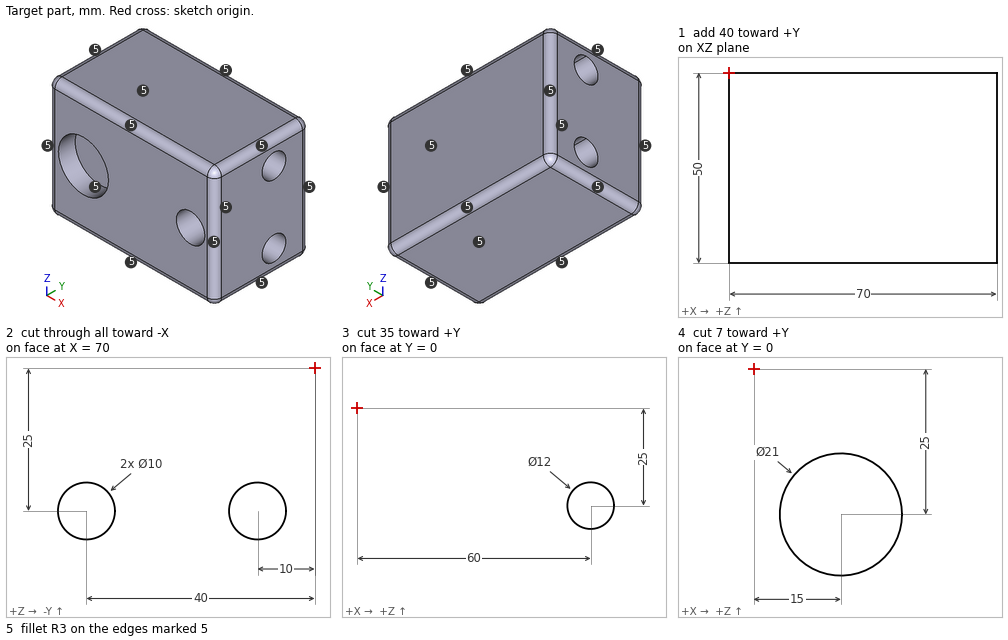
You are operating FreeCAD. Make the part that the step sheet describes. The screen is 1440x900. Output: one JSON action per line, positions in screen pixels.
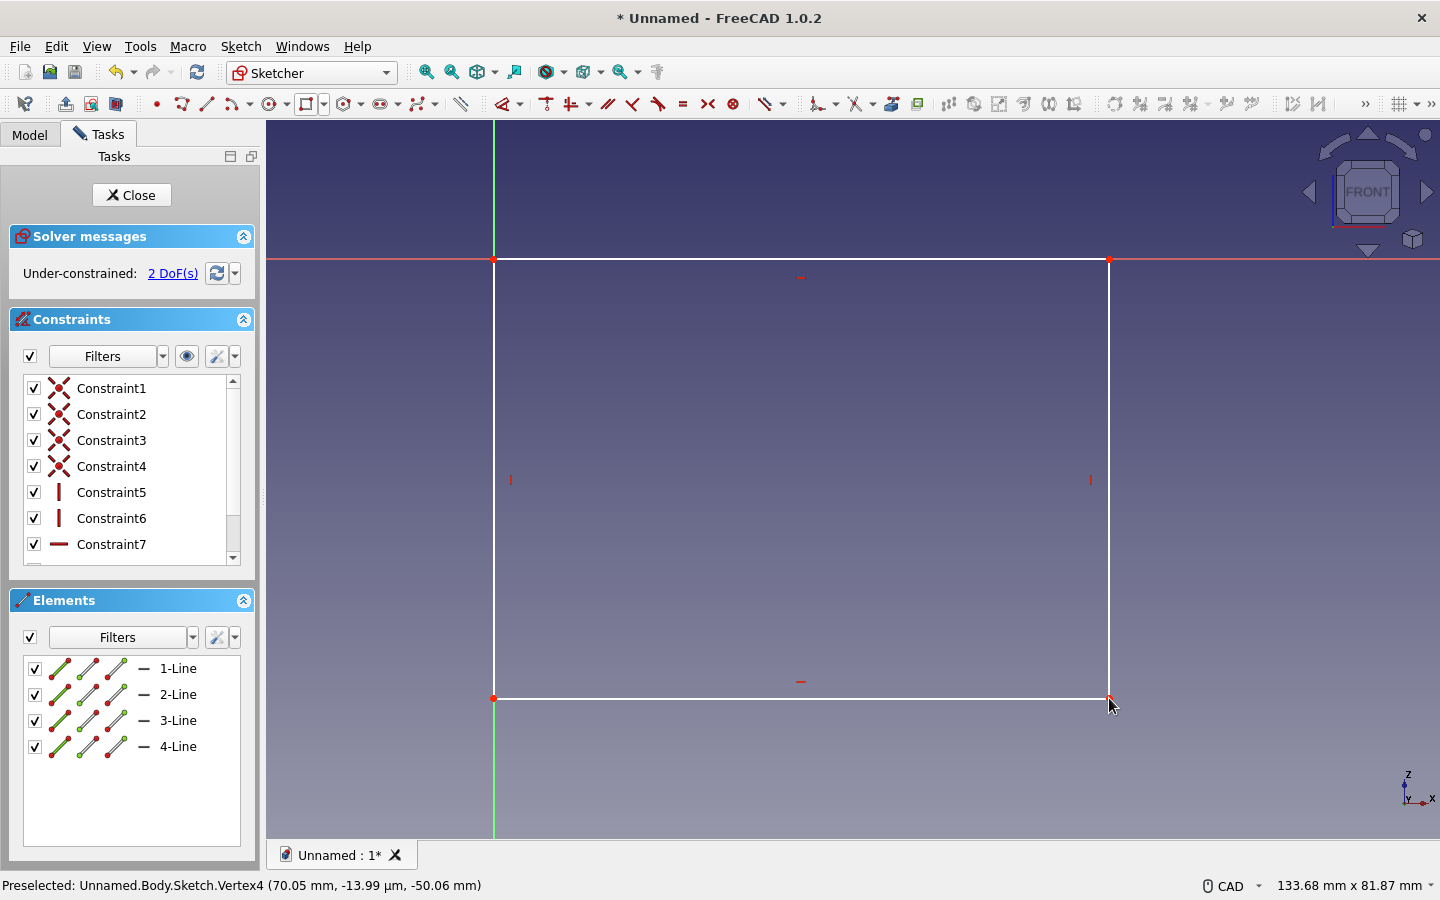
{"action": "left_click", "coordinate": [494, 391]}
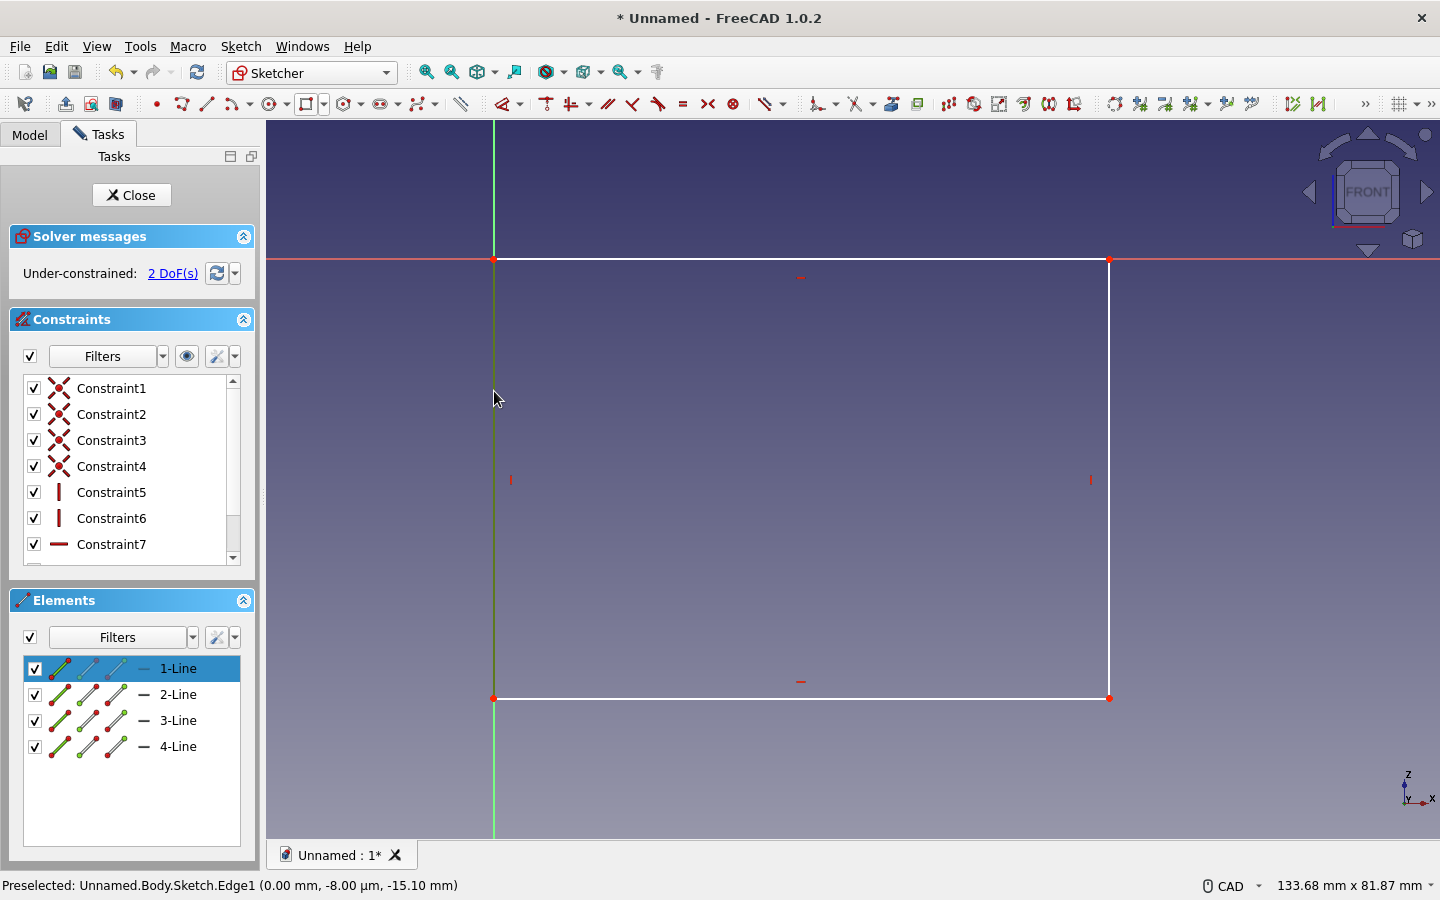
{"action": "key", "text": "i"}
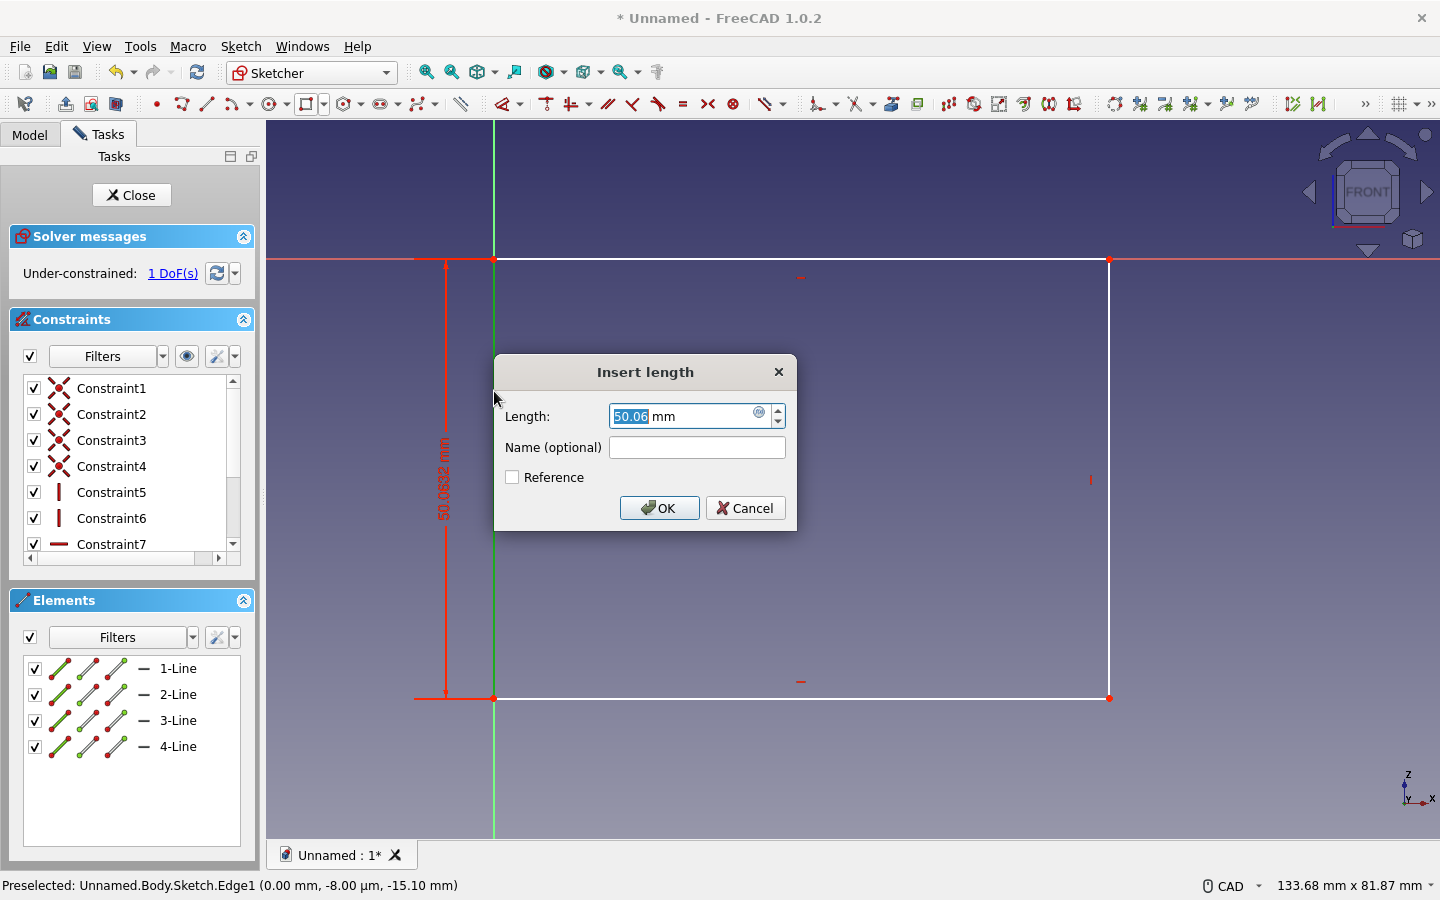
{"action": "type", "text": "50"}
{"action": "key", "text": "Return"}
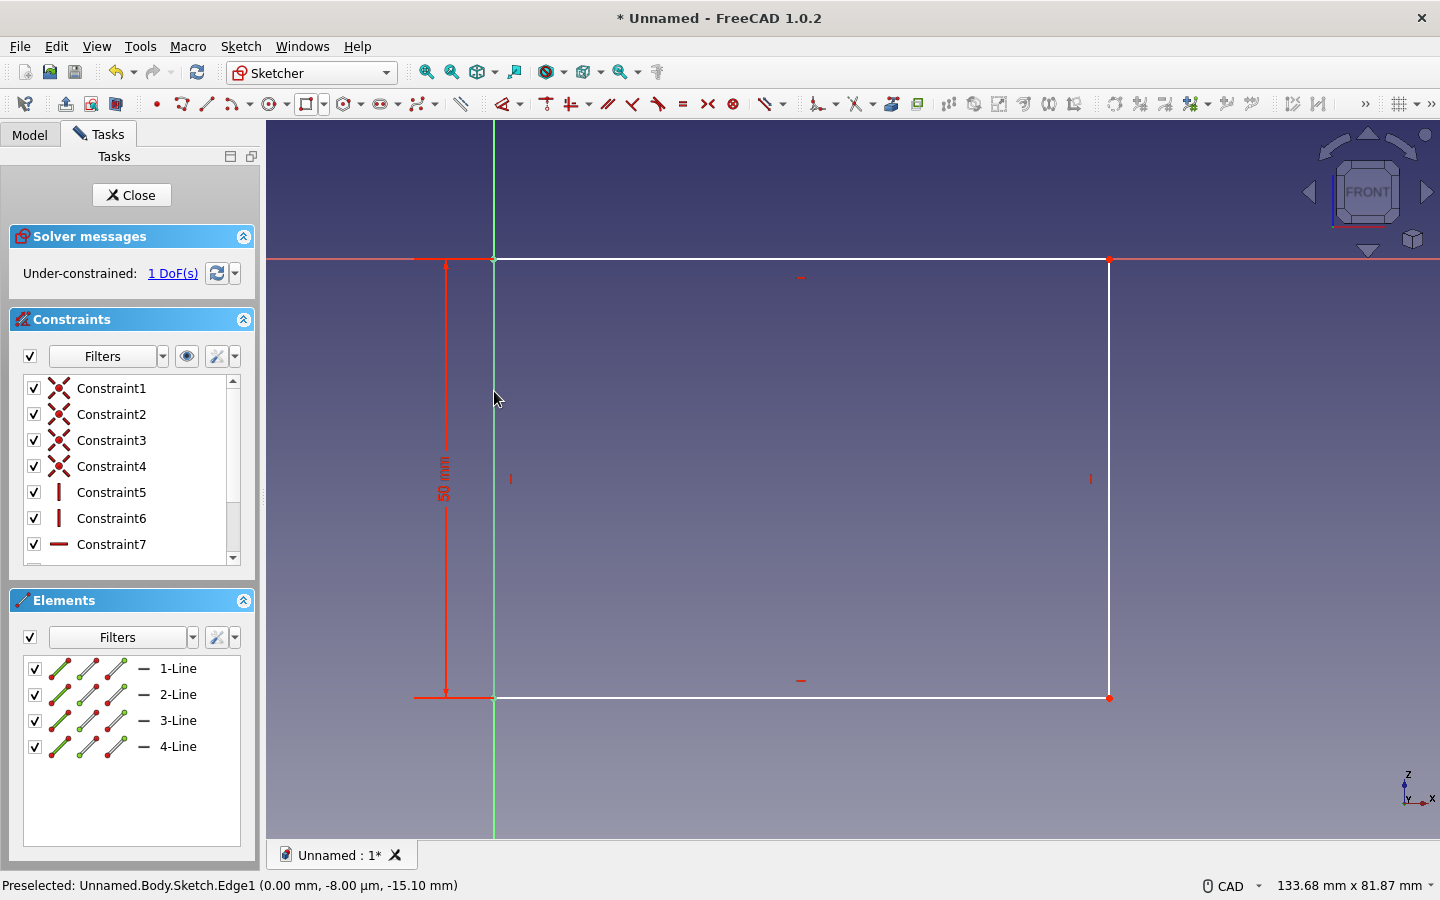
{"action": "left_click", "coordinate": [678, 698]}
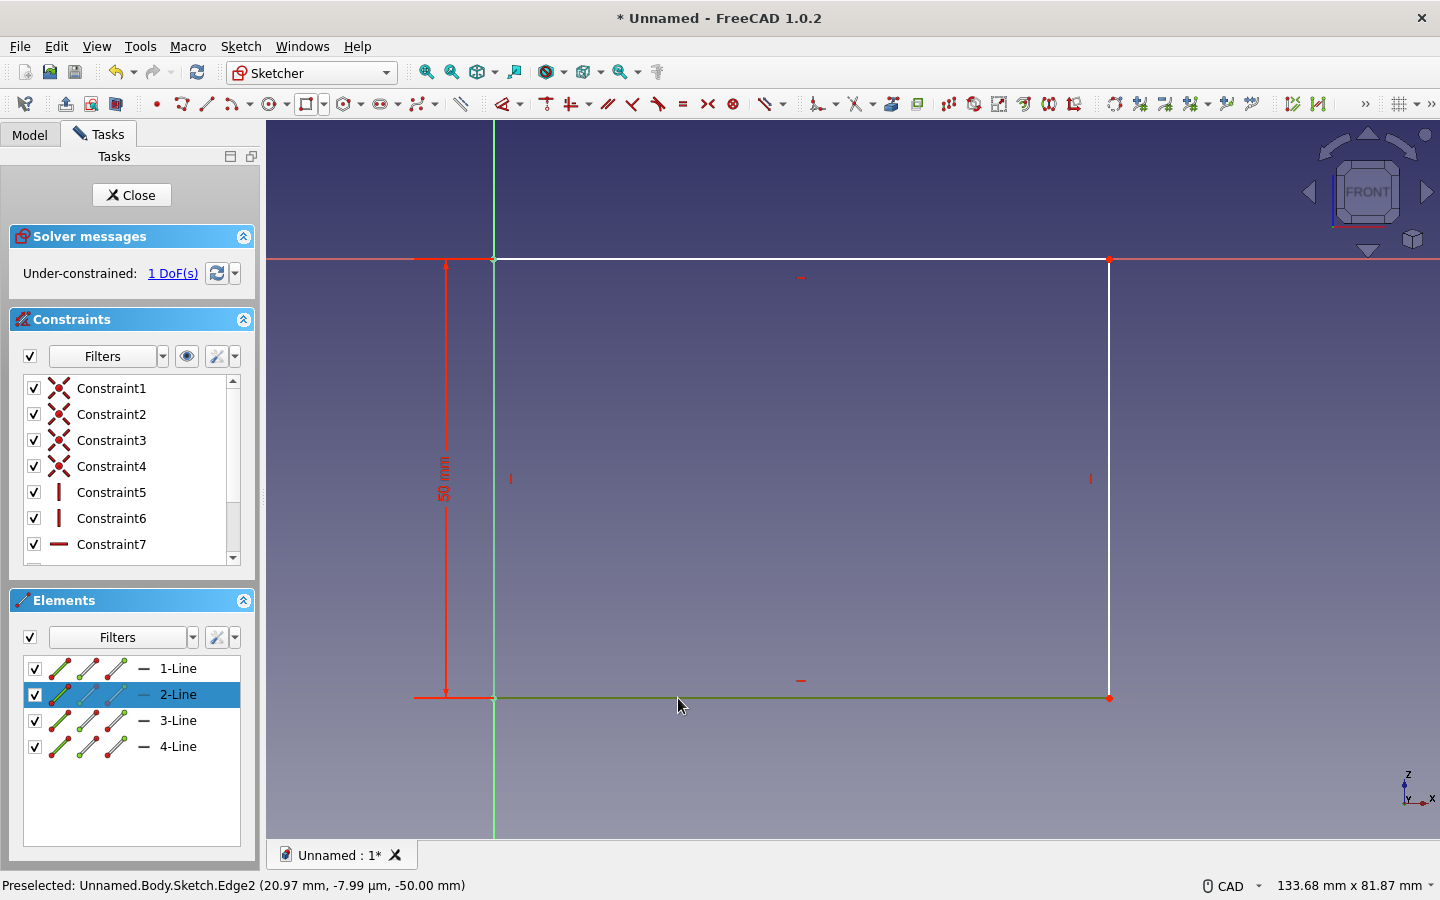
{"action": "key", "text": "l"}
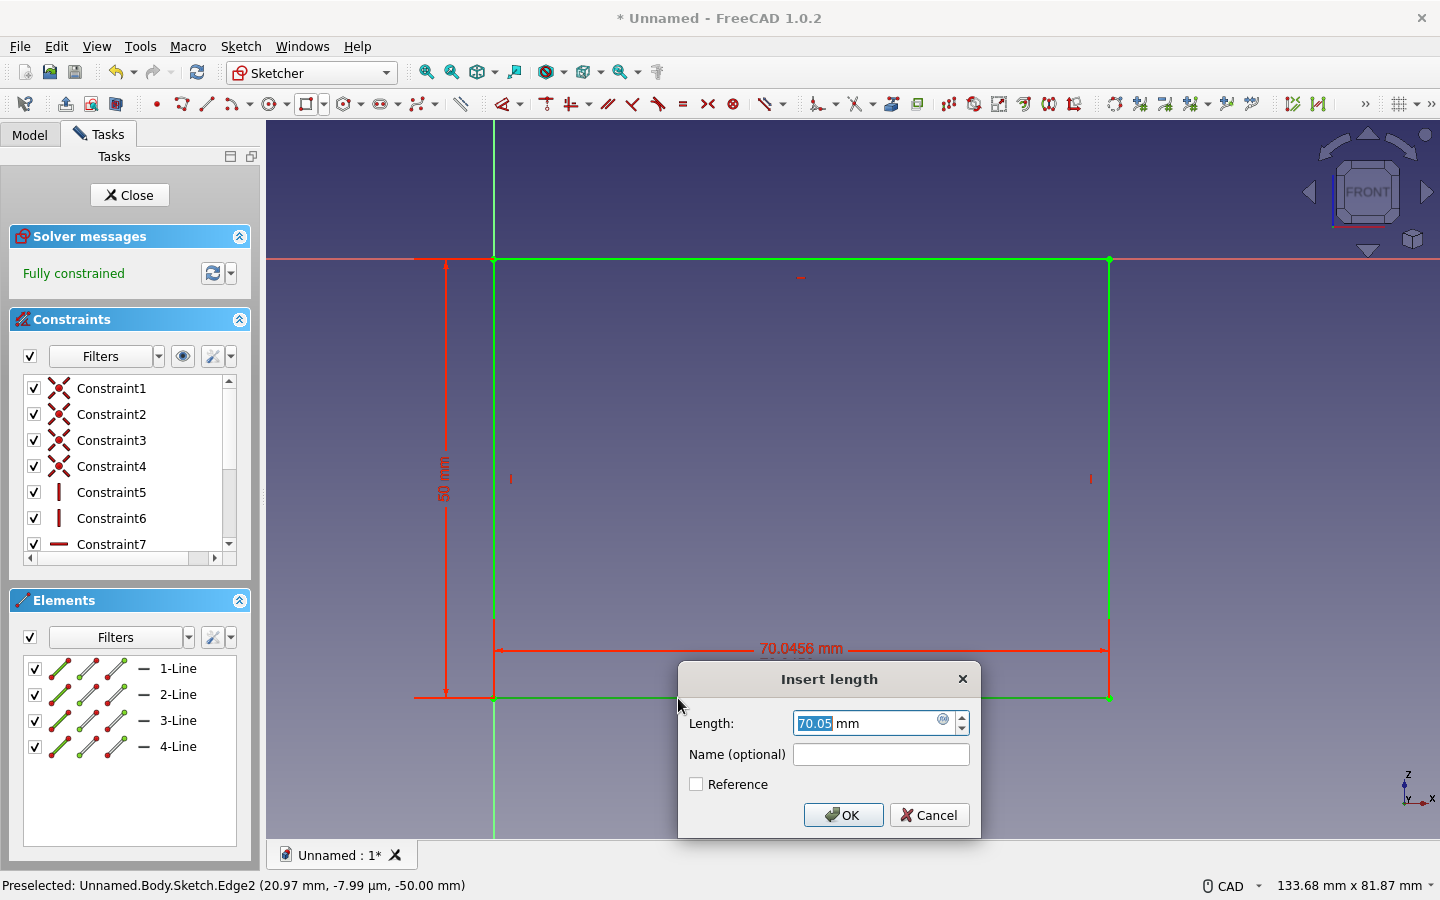
{"action": "type", "text": "70"}
{"action": "key", "text": "Return"}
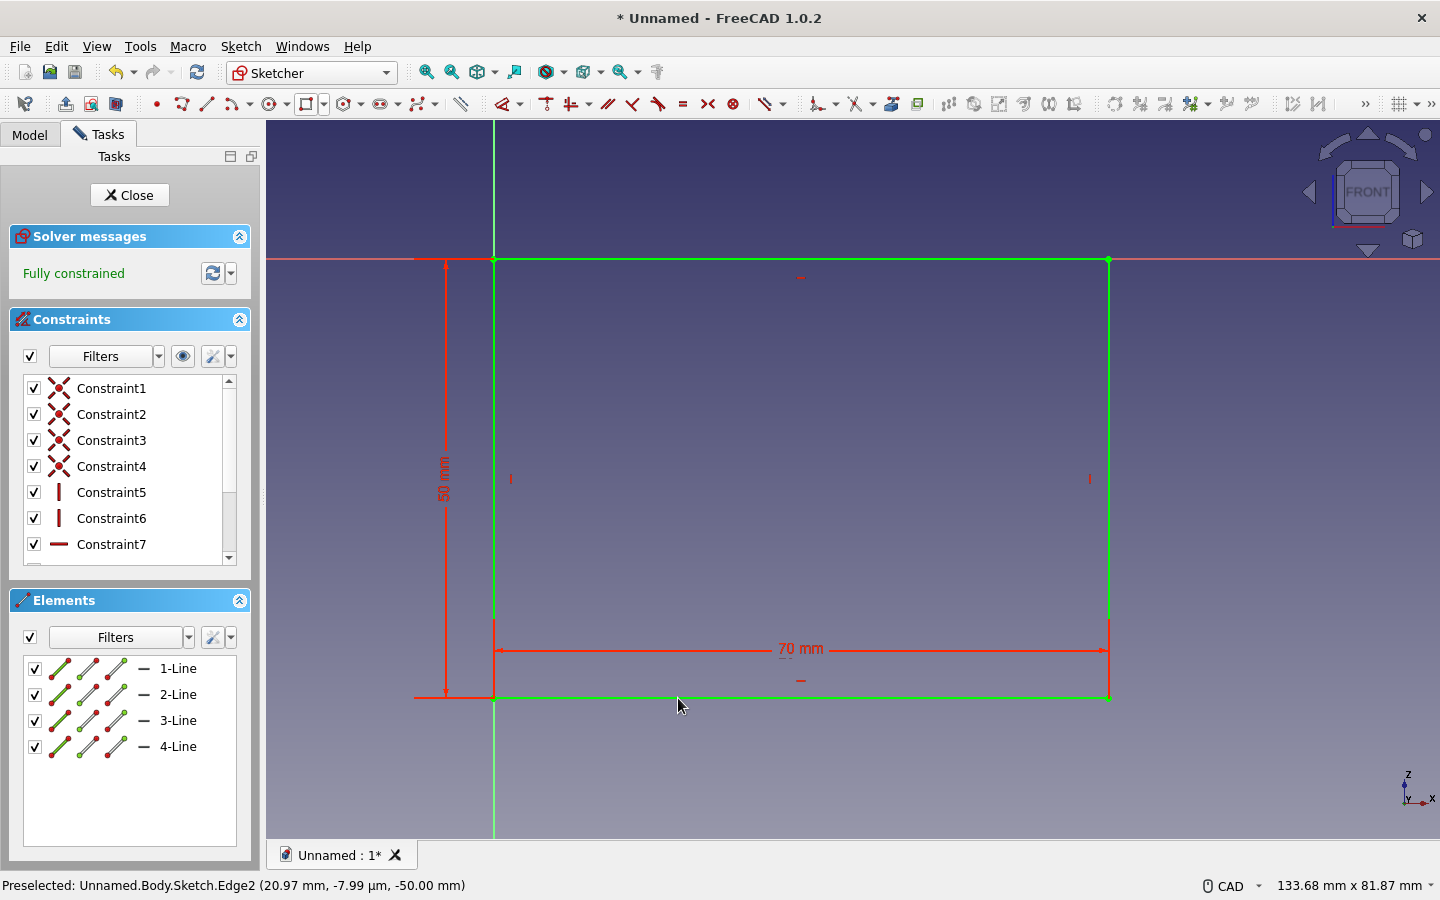
{"action": "left_click", "coordinate": [130, 195]}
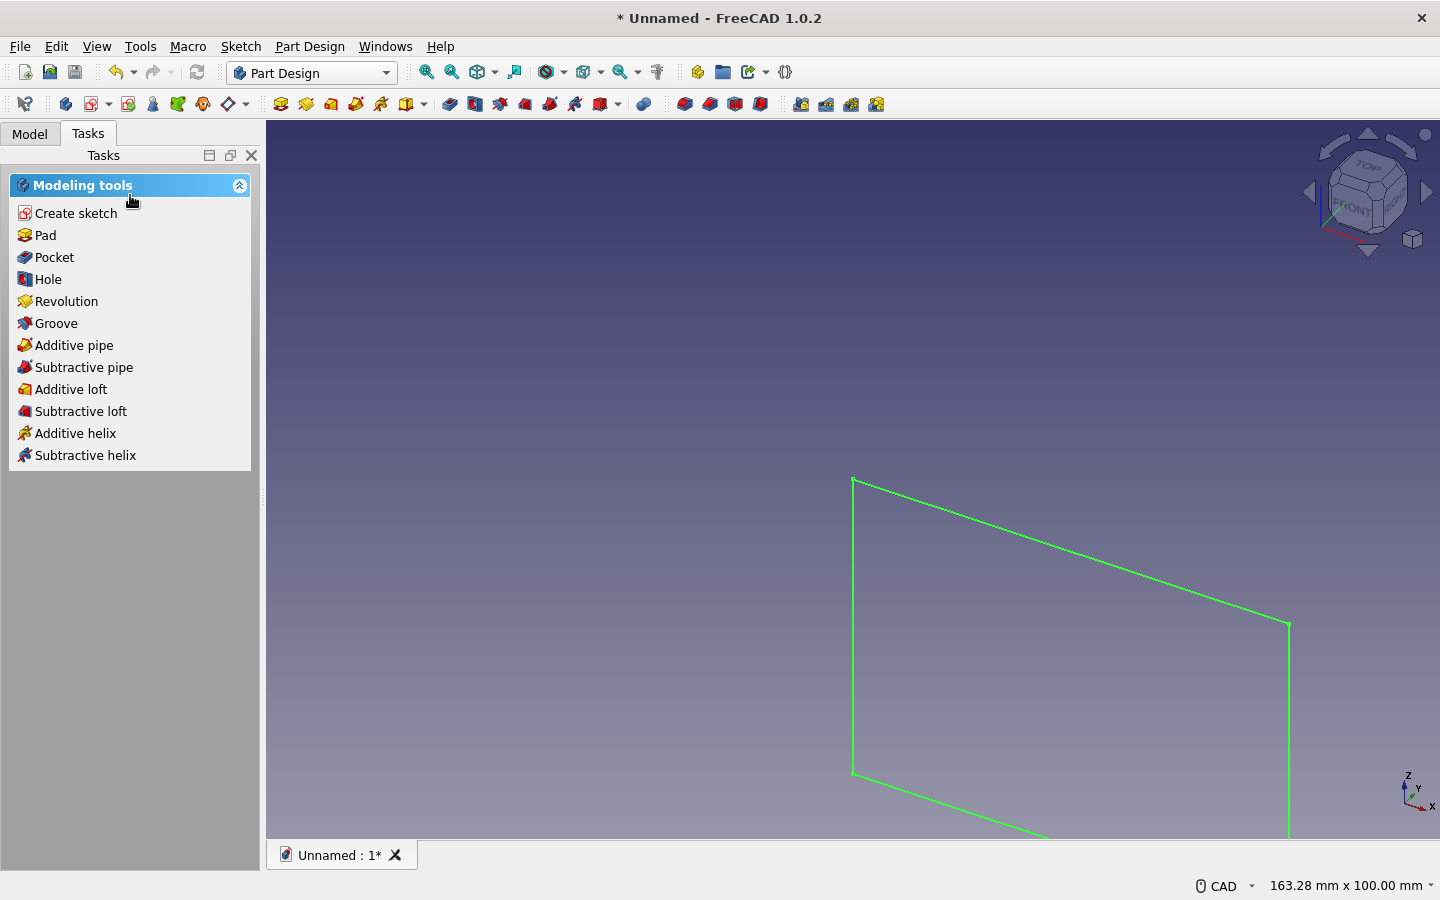
{"action": "left_click", "coordinate": [281, 104]}